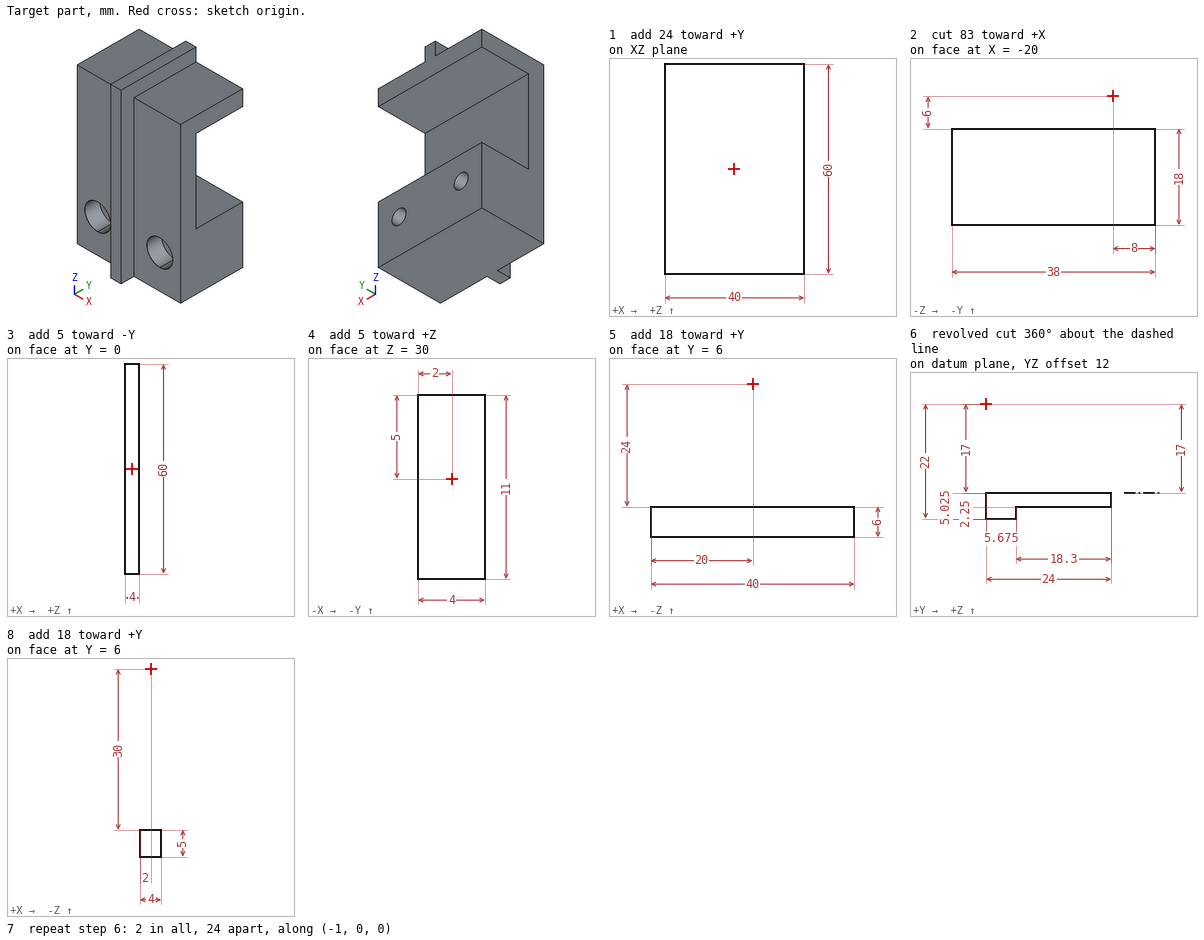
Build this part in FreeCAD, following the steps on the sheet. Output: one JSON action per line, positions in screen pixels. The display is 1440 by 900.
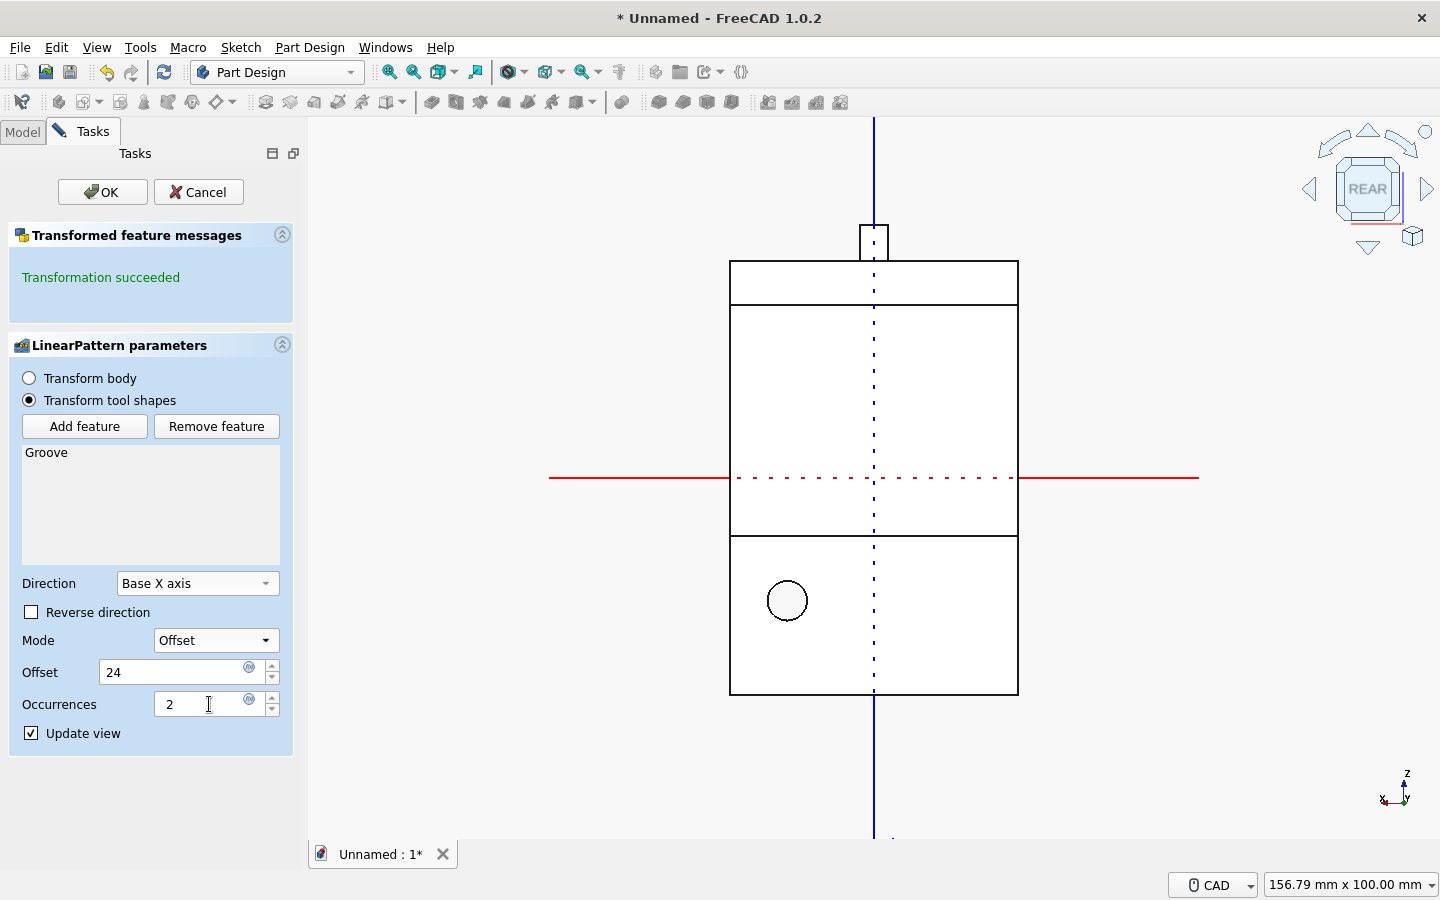
{"action": "left_click", "coordinate": [30, 612]}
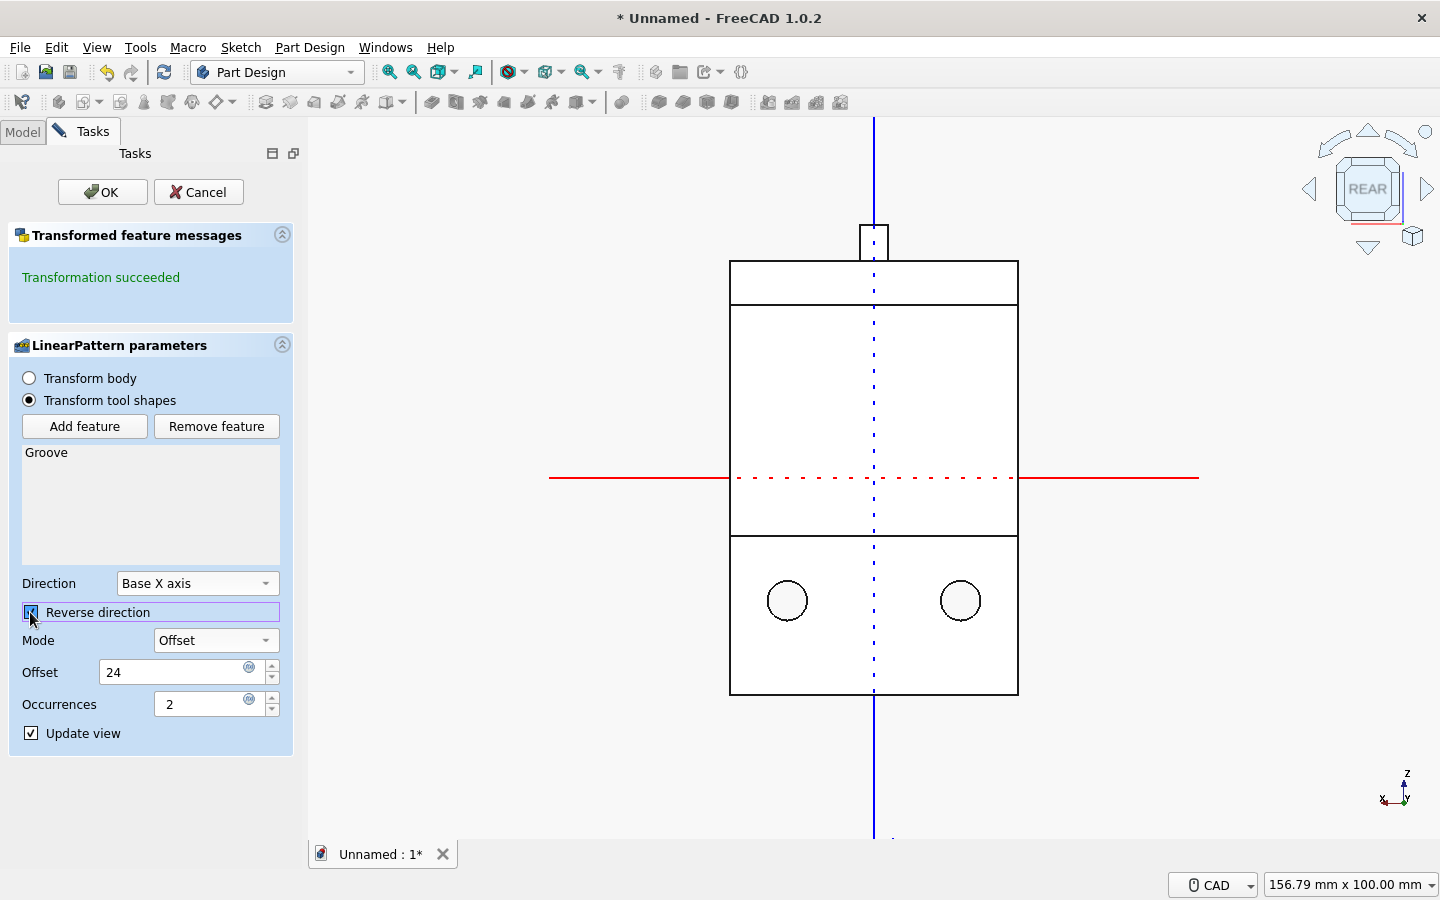
{"action": "left_click", "coordinate": [103, 192]}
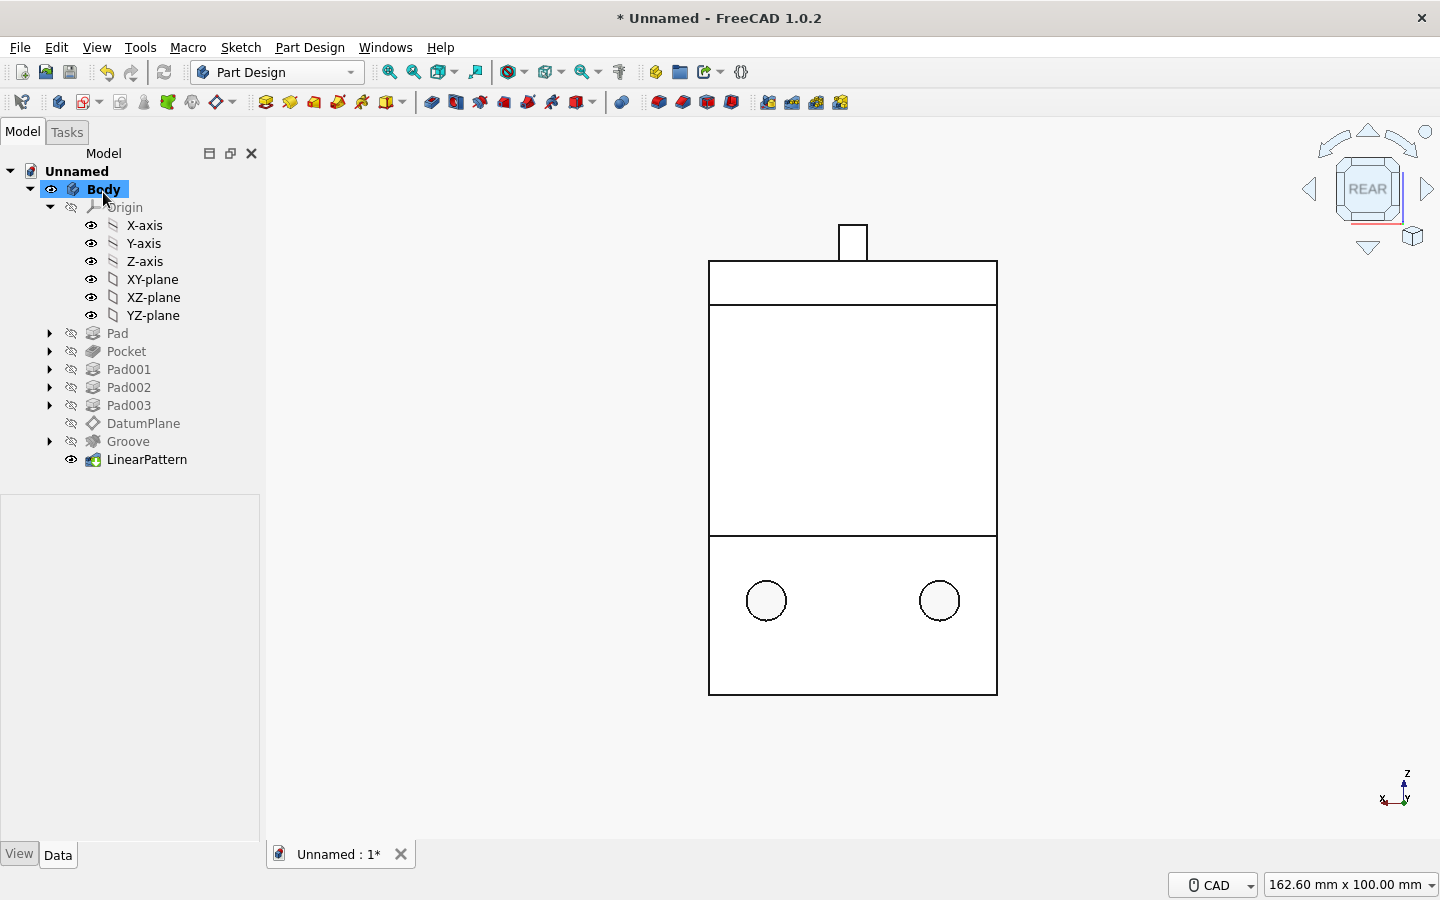
{"action": "left_click", "coordinate": [853, 419]}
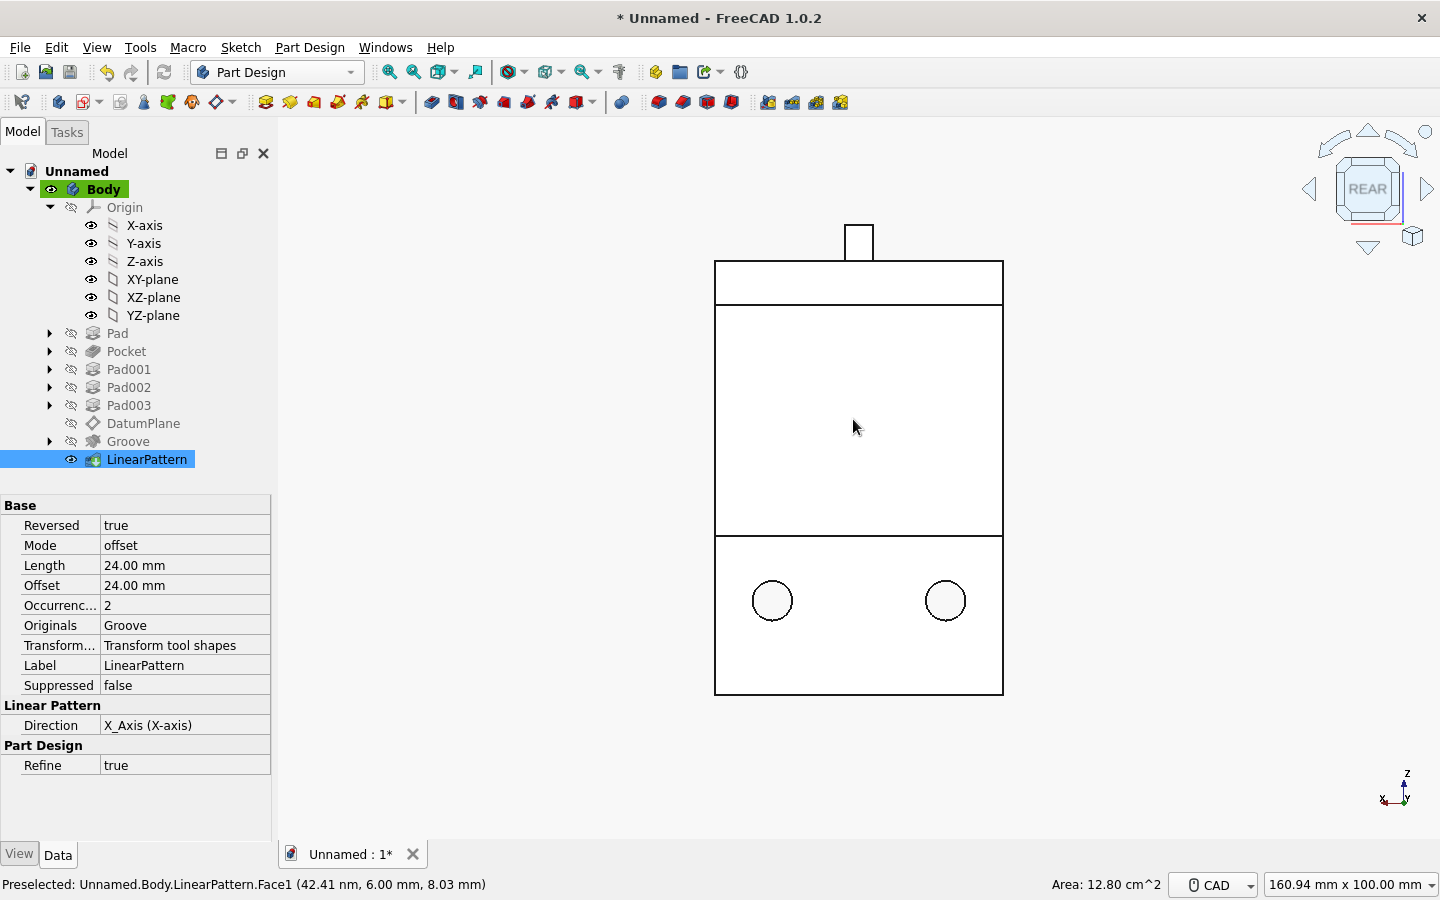
{"action": "left_click", "coordinate": [84, 102]}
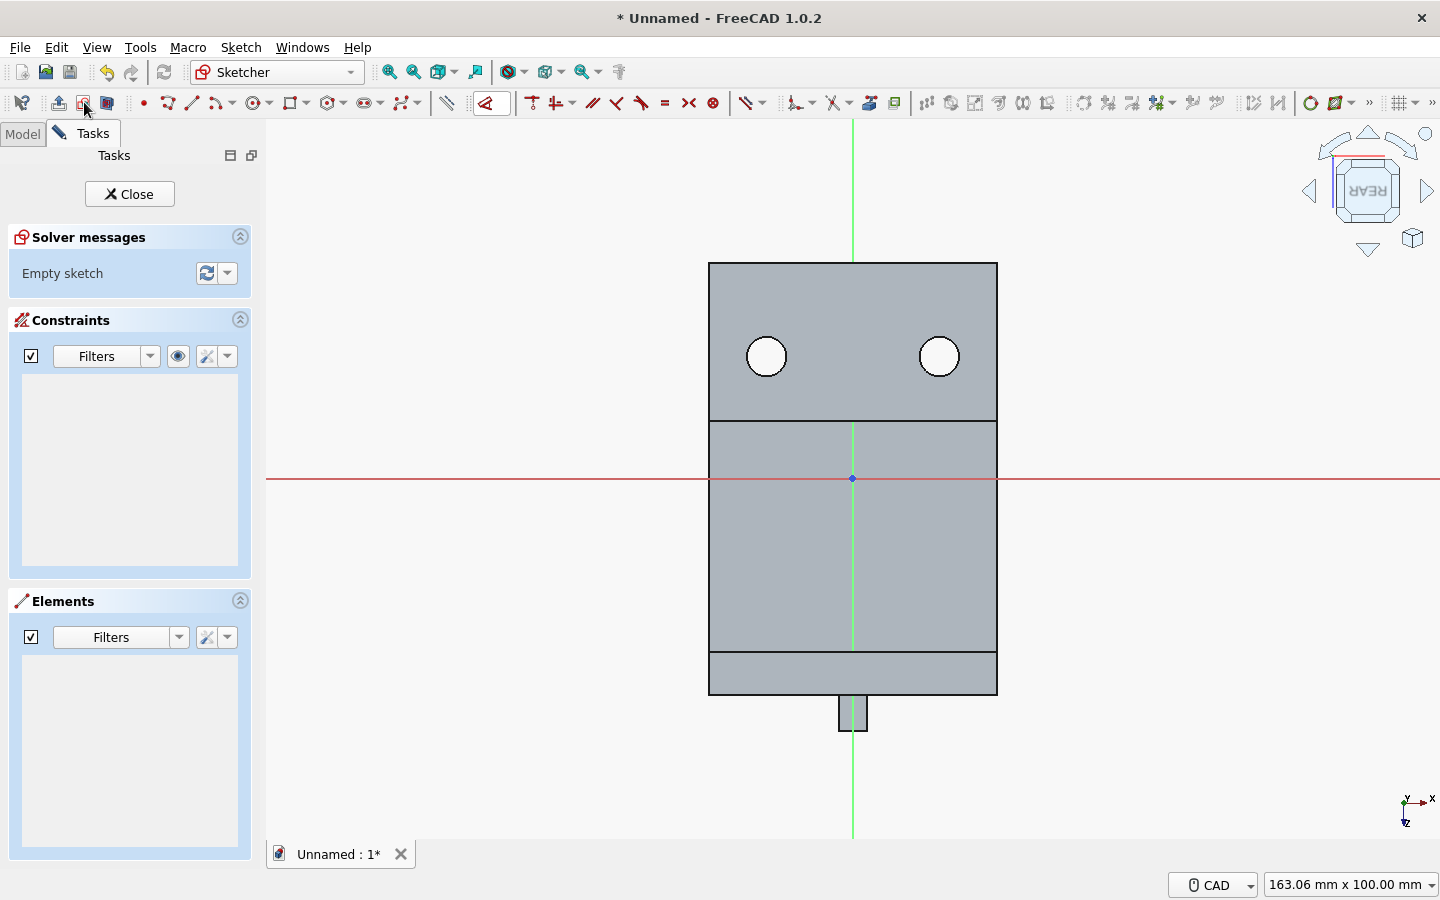
{"action": "key", "text": "q s"}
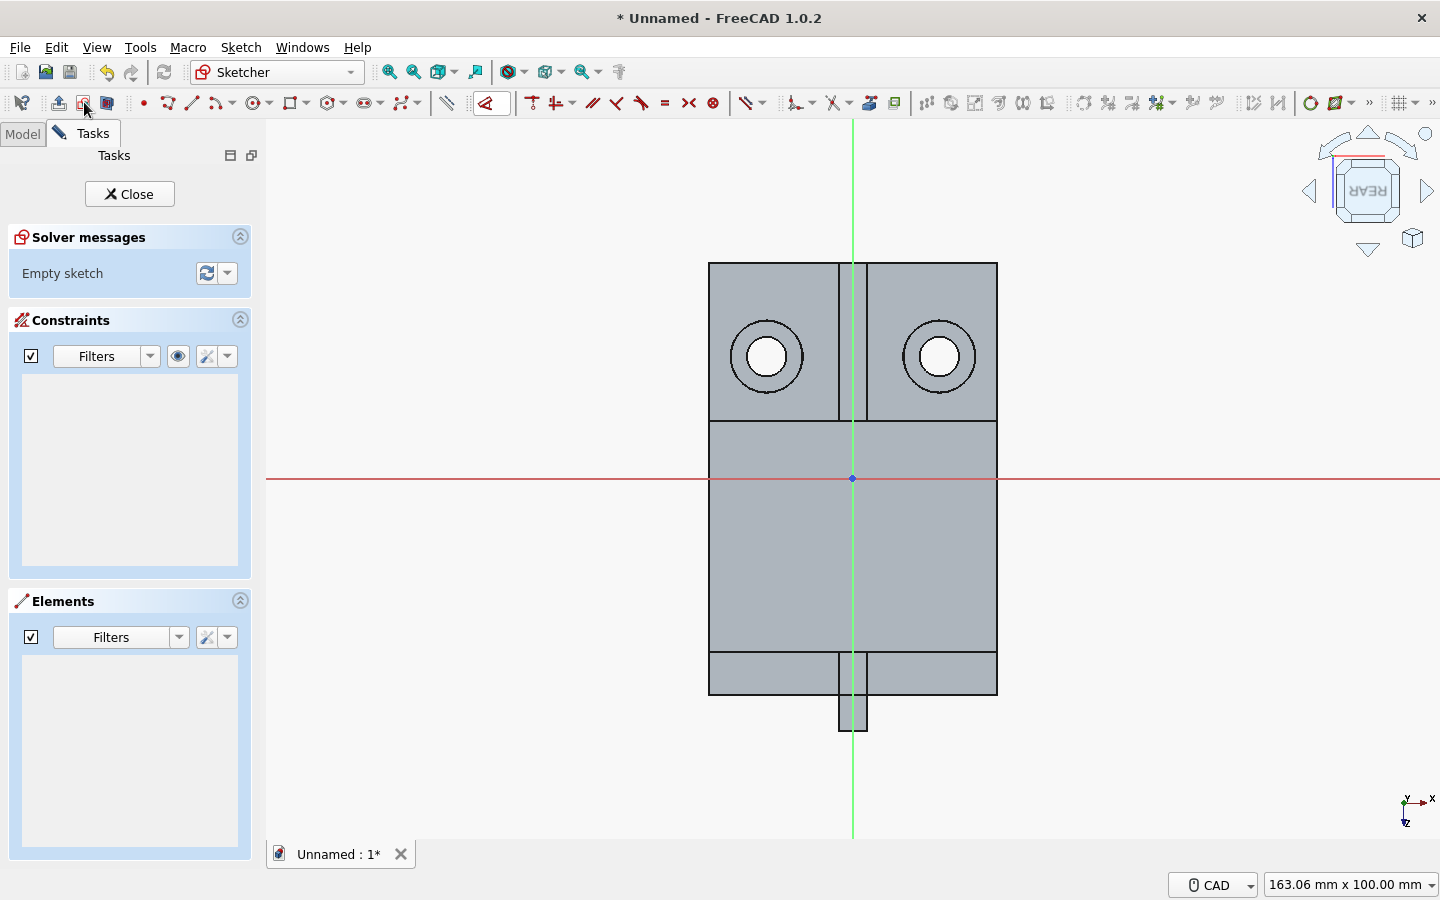
{"action": "scroll", "coordinate": [858, 732], "scroll_direction": "up", "scroll_amount": 13}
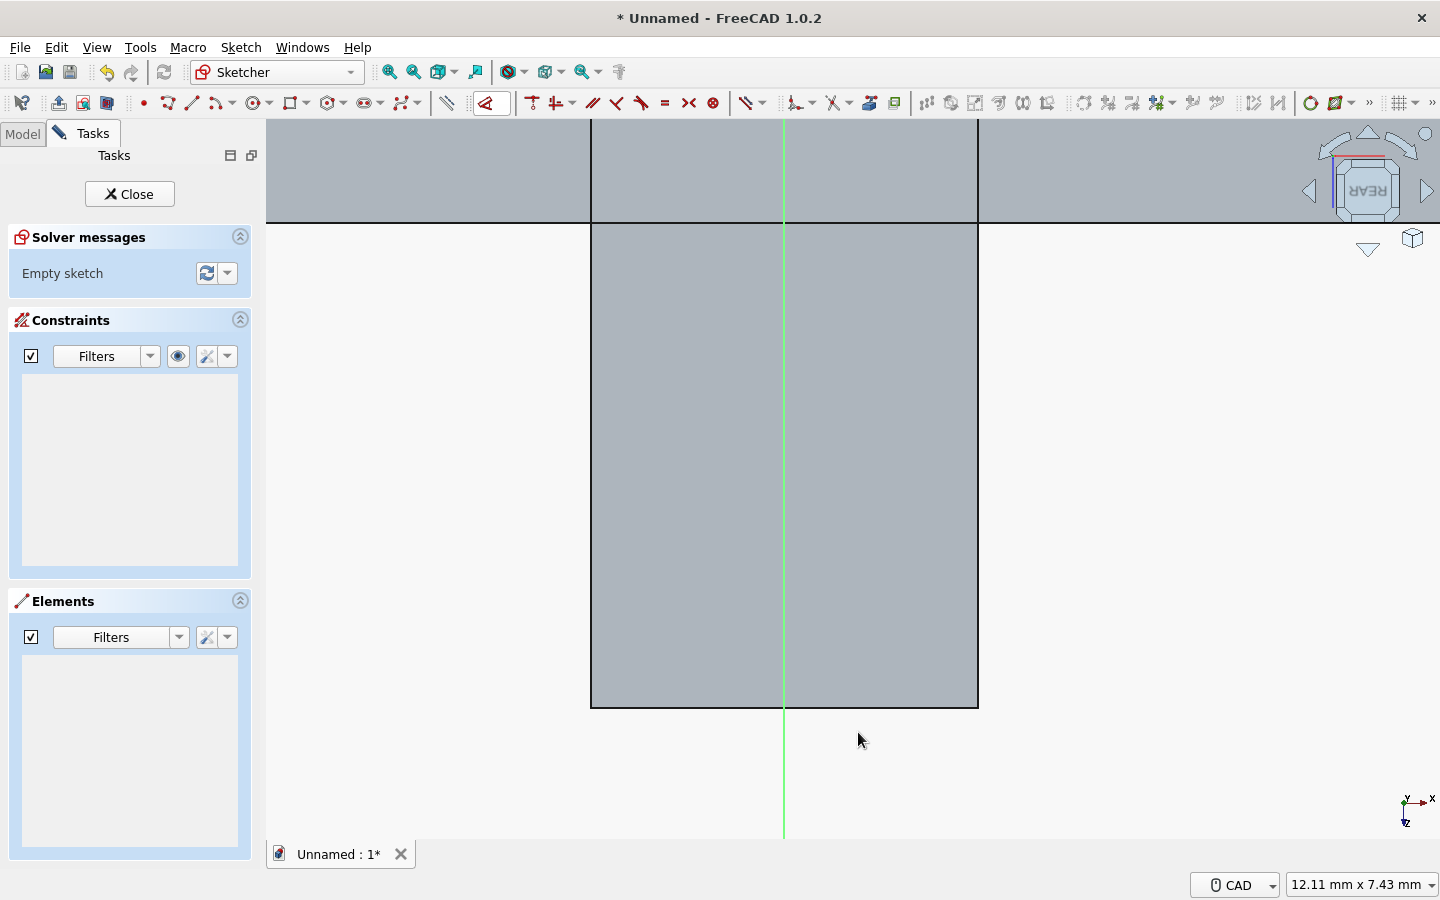
{"action": "left_click", "coordinate": [290, 104]}